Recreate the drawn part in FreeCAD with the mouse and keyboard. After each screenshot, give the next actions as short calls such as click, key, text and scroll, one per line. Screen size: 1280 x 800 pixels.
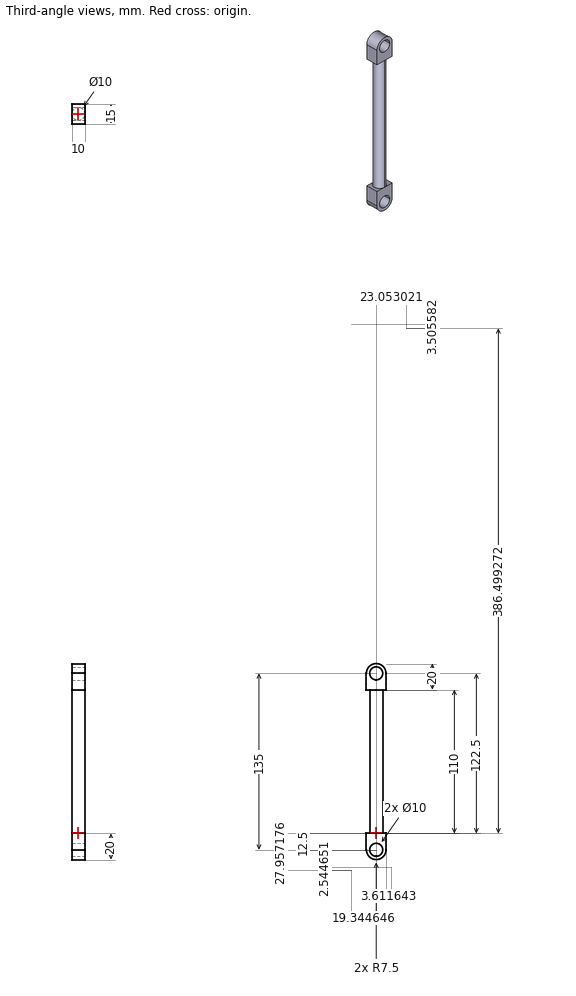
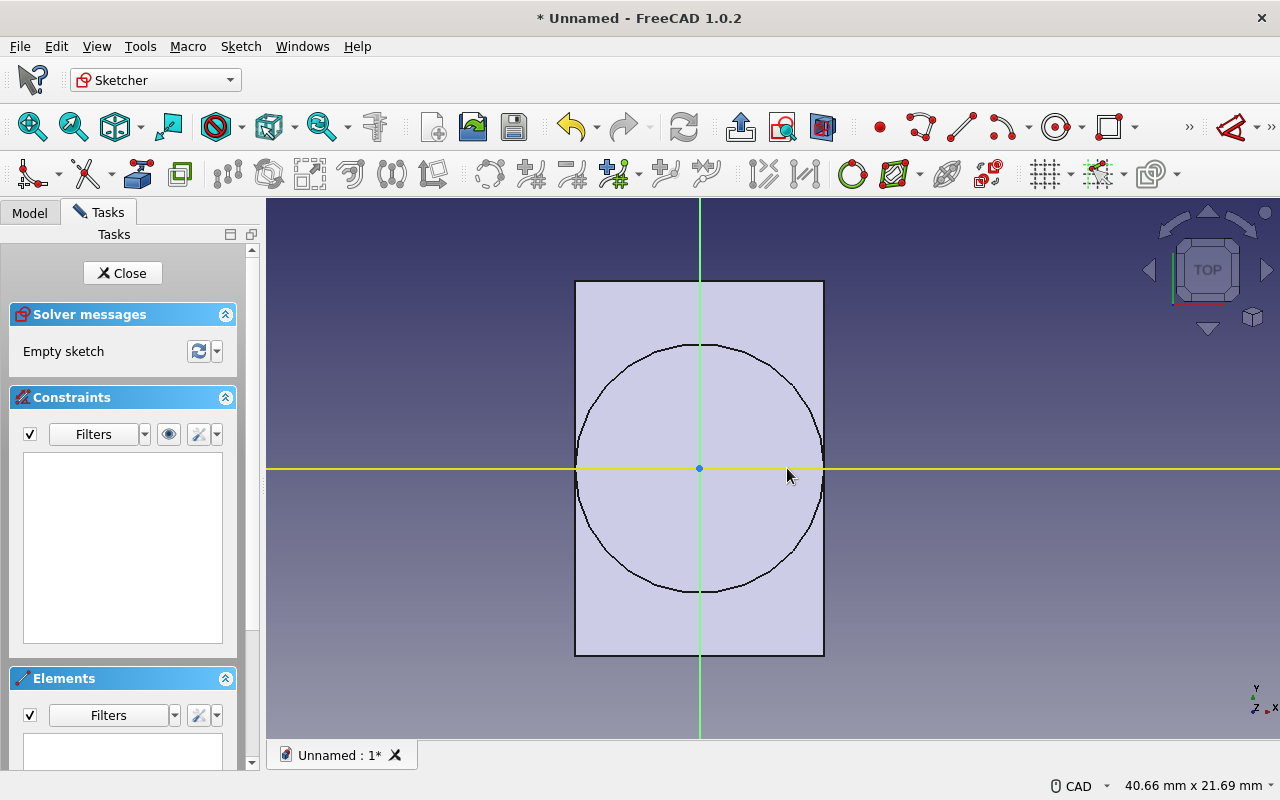
click(1134, 128)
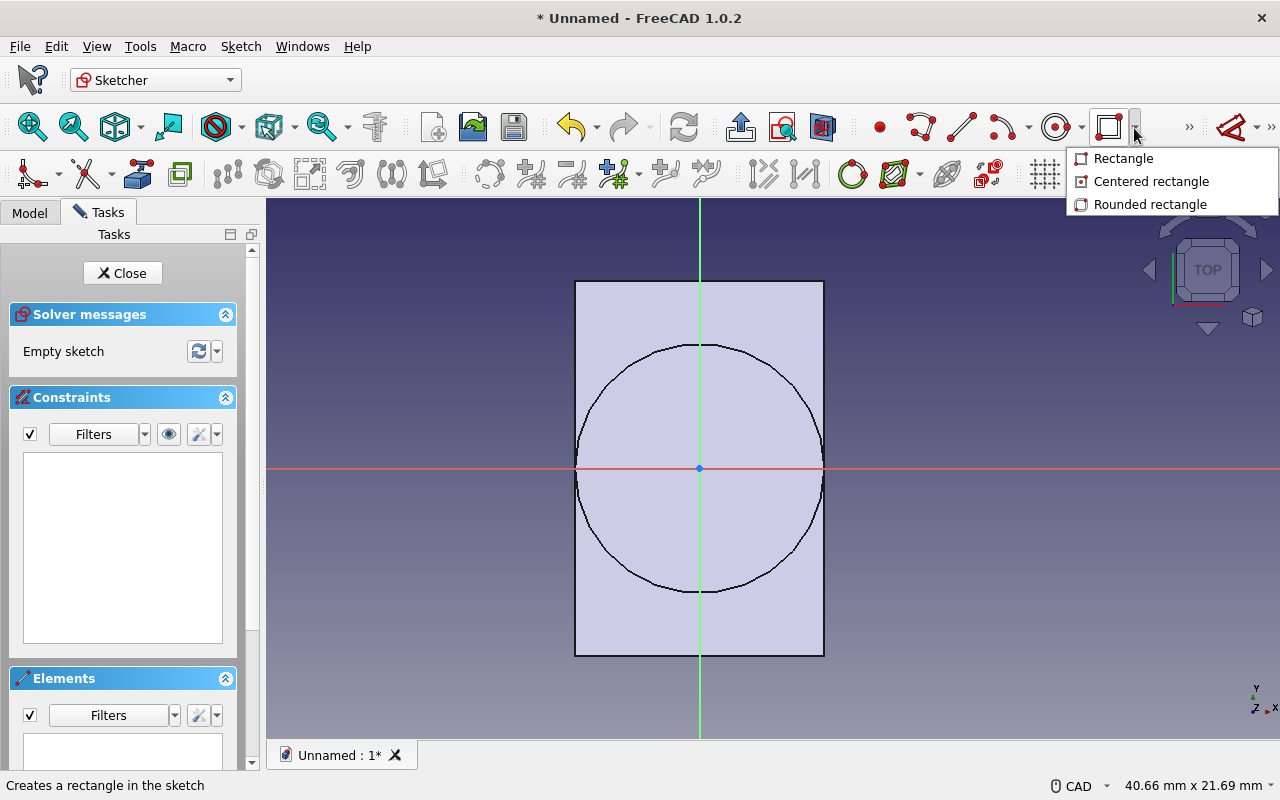
click(1172, 182)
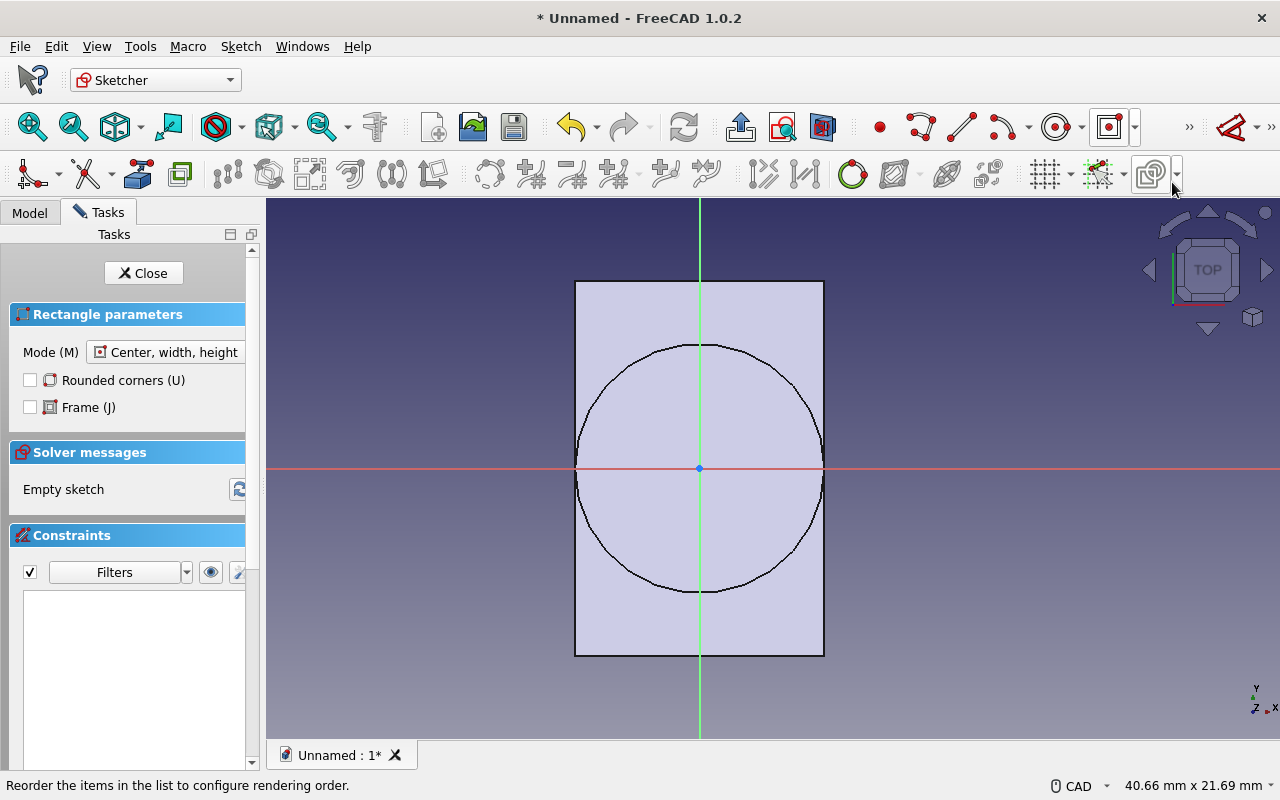
click(700, 468)
move(824, 281)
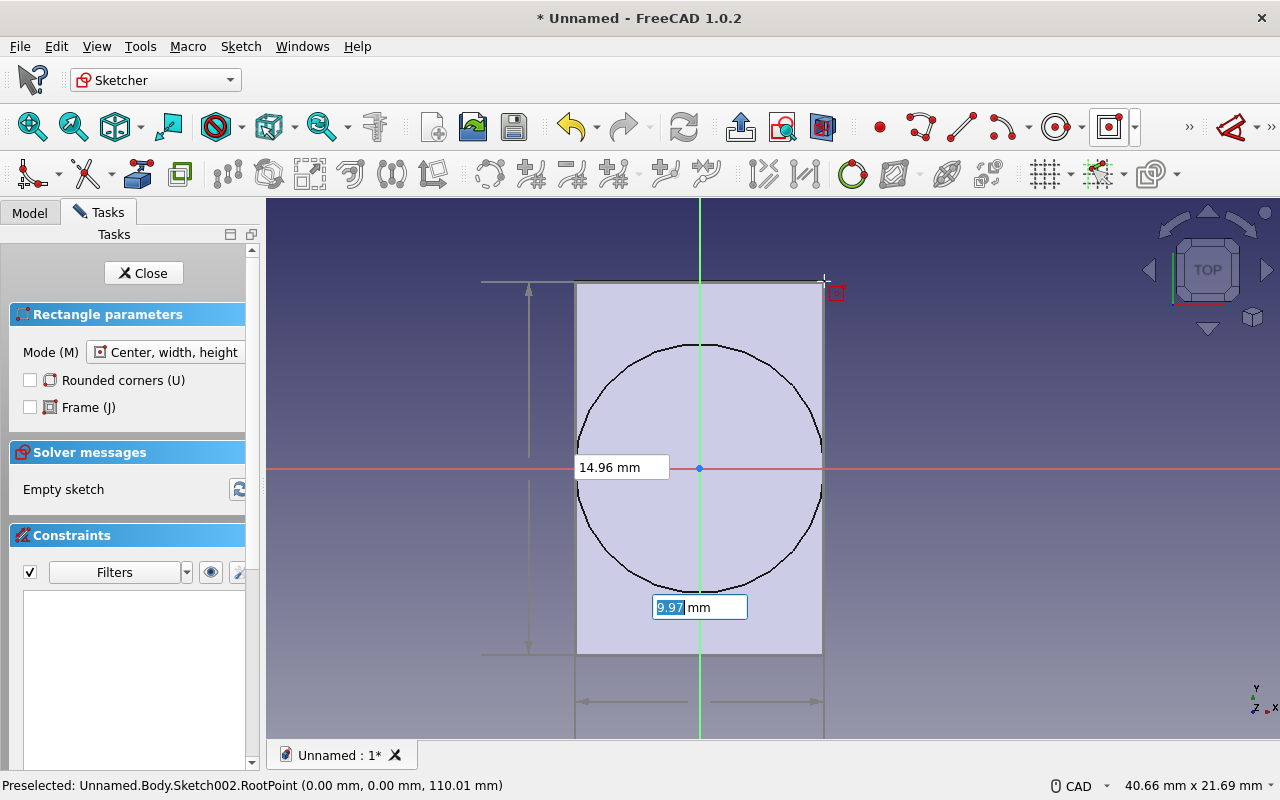
text(10)
key(Tab)
text(15)
key(Return)
key(Escape)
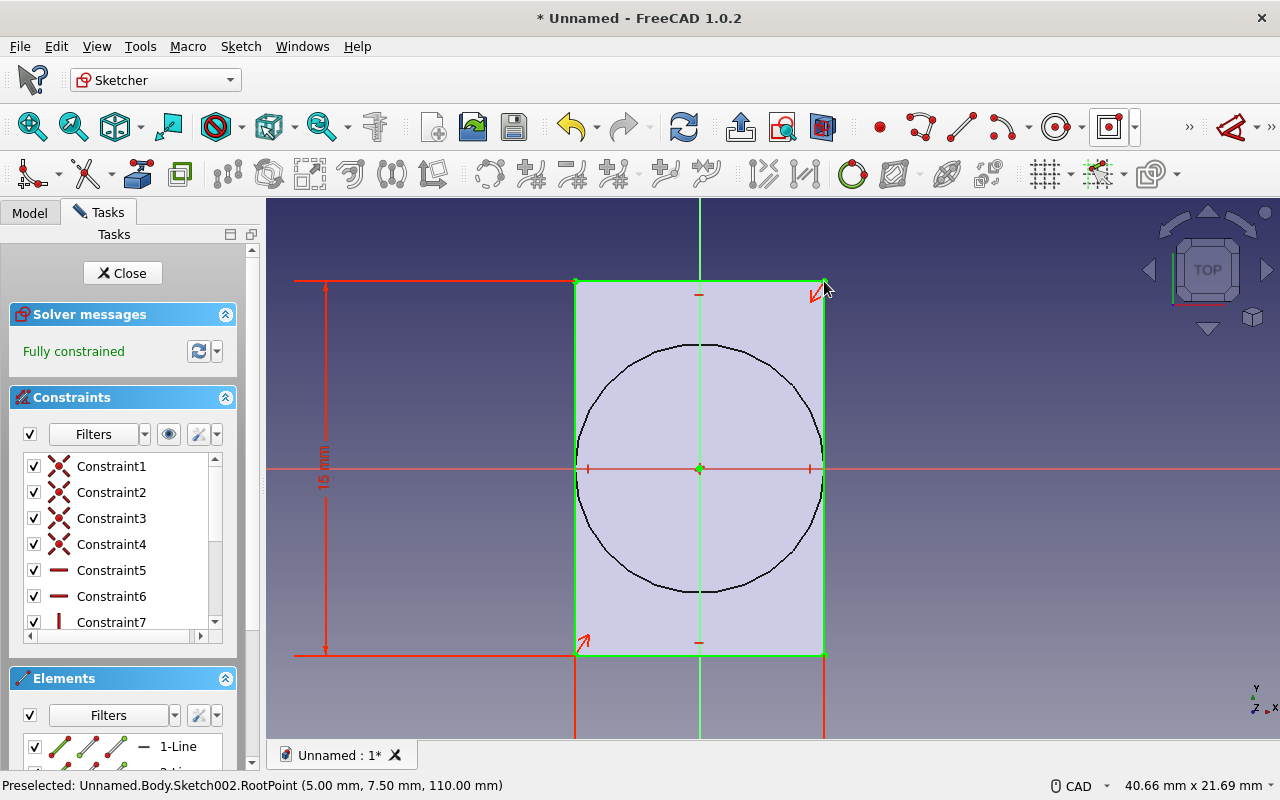
click(123, 273)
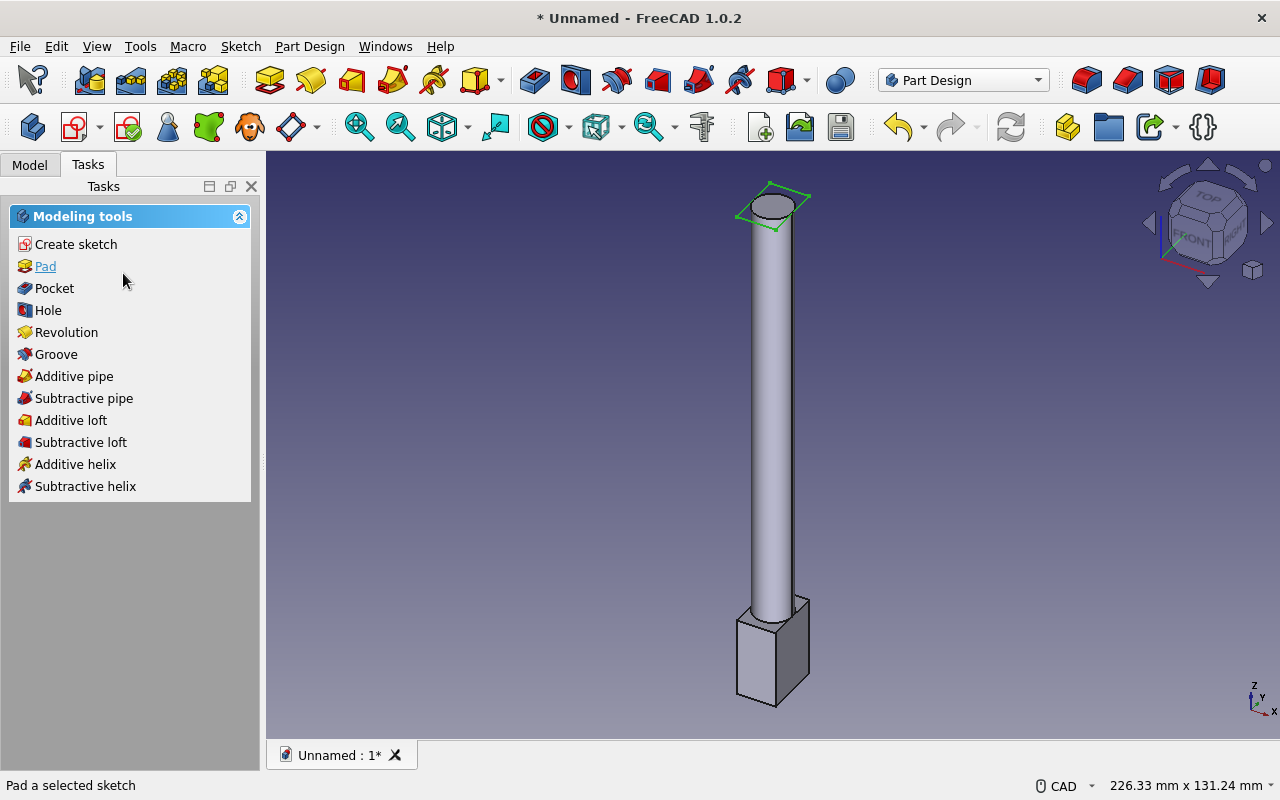
click(270, 80)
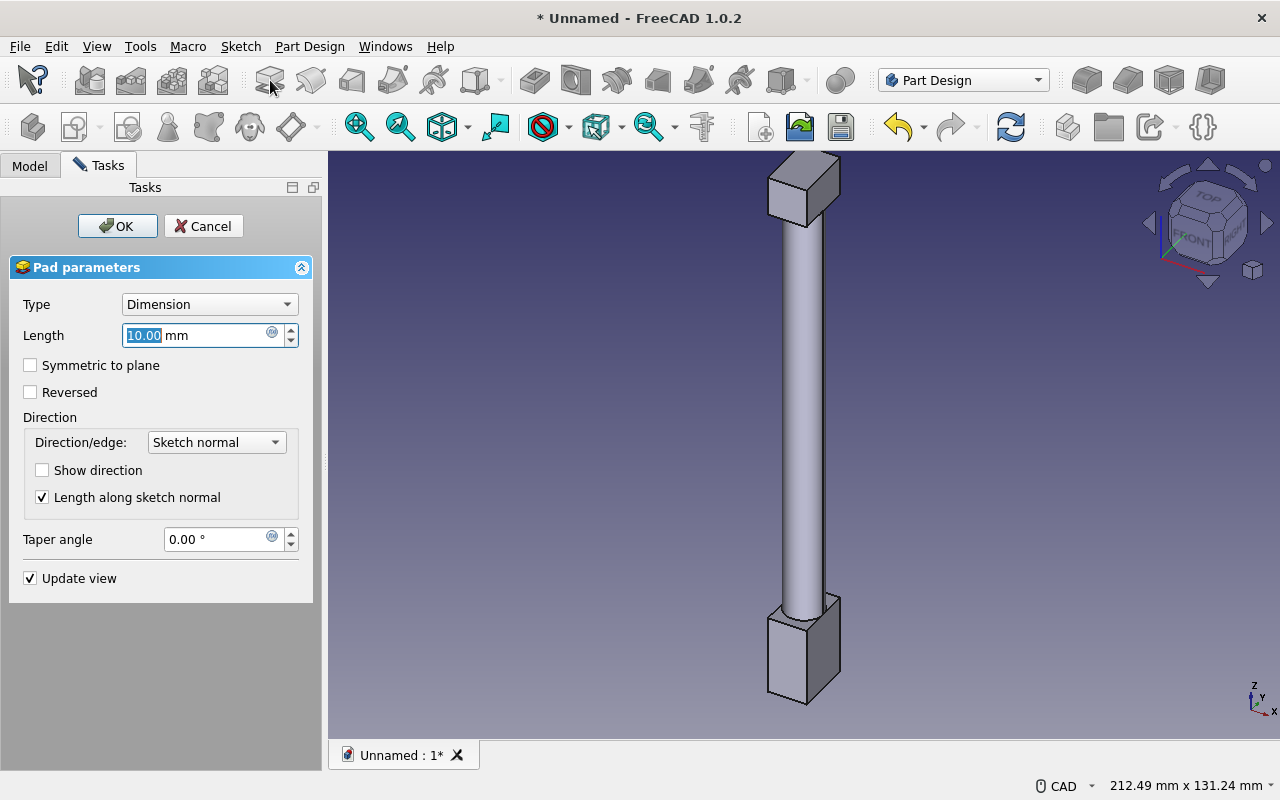
text(20)
key(Tab)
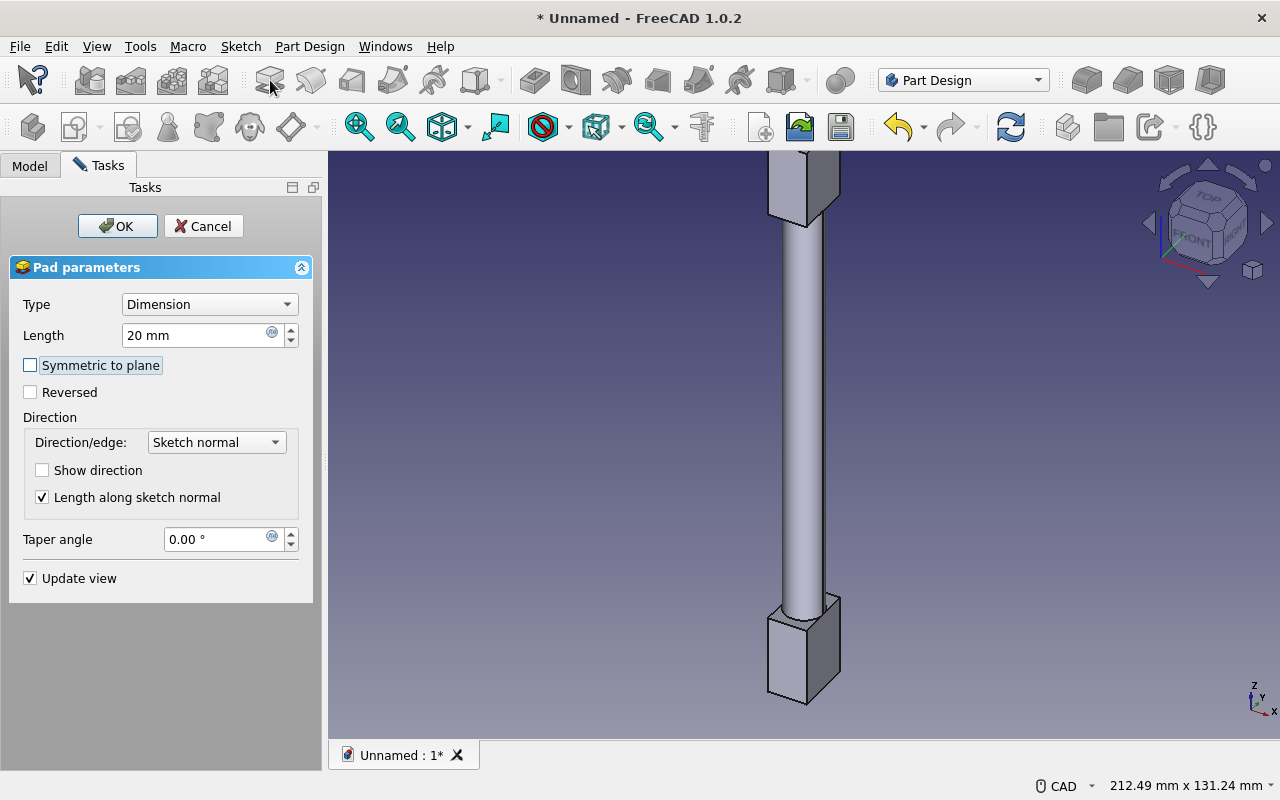
click(118, 226)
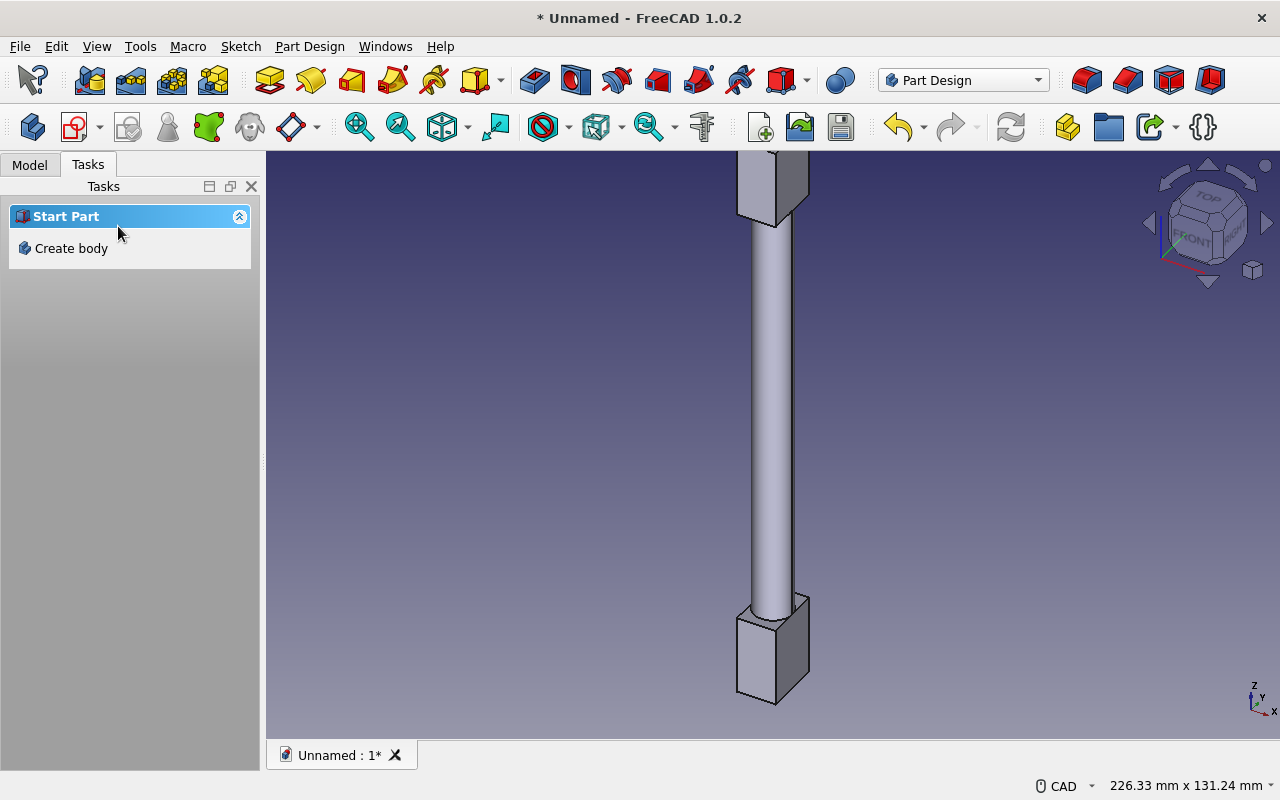
click(360, 128)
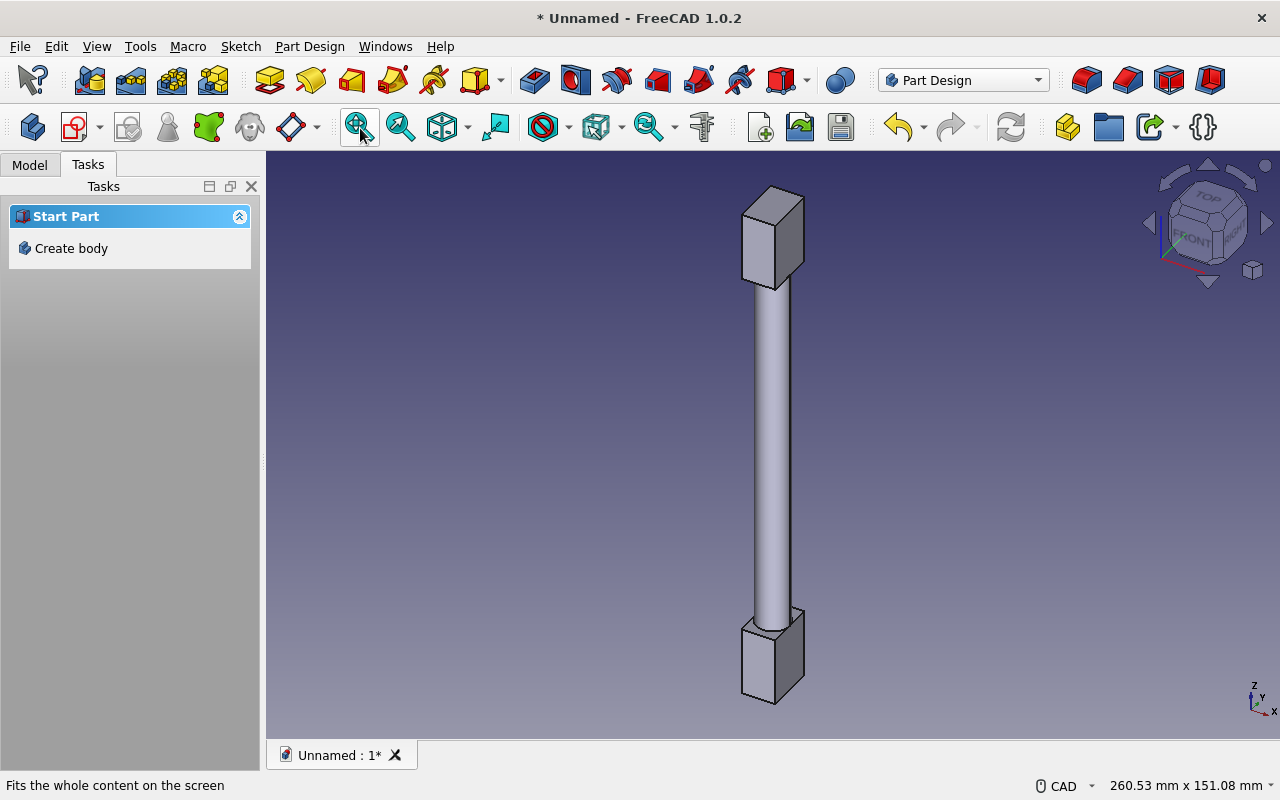
click(790, 242)